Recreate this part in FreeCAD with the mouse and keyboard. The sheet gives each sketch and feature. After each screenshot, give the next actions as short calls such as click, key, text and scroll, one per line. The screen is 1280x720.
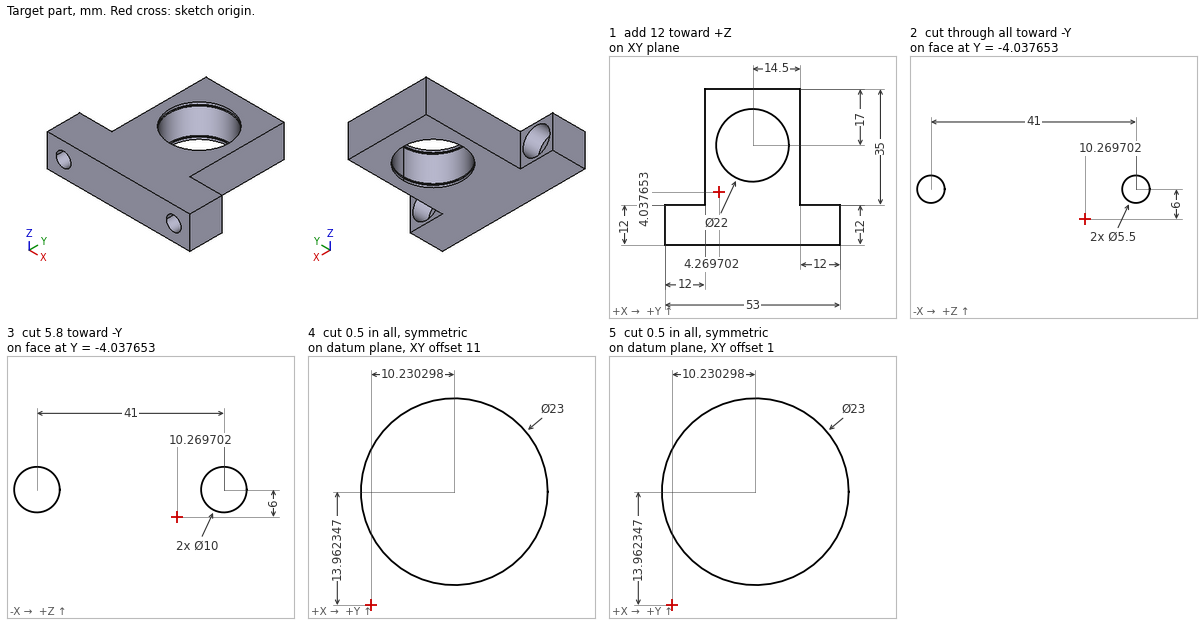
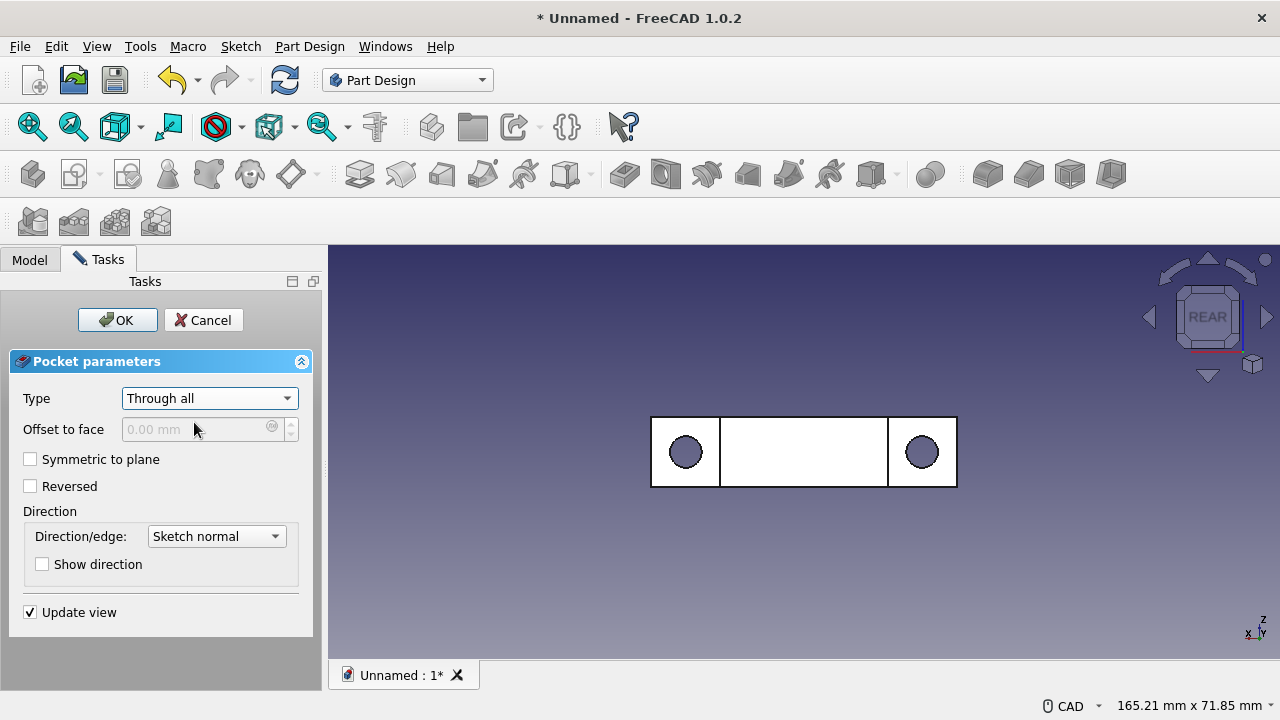
click(118, 320)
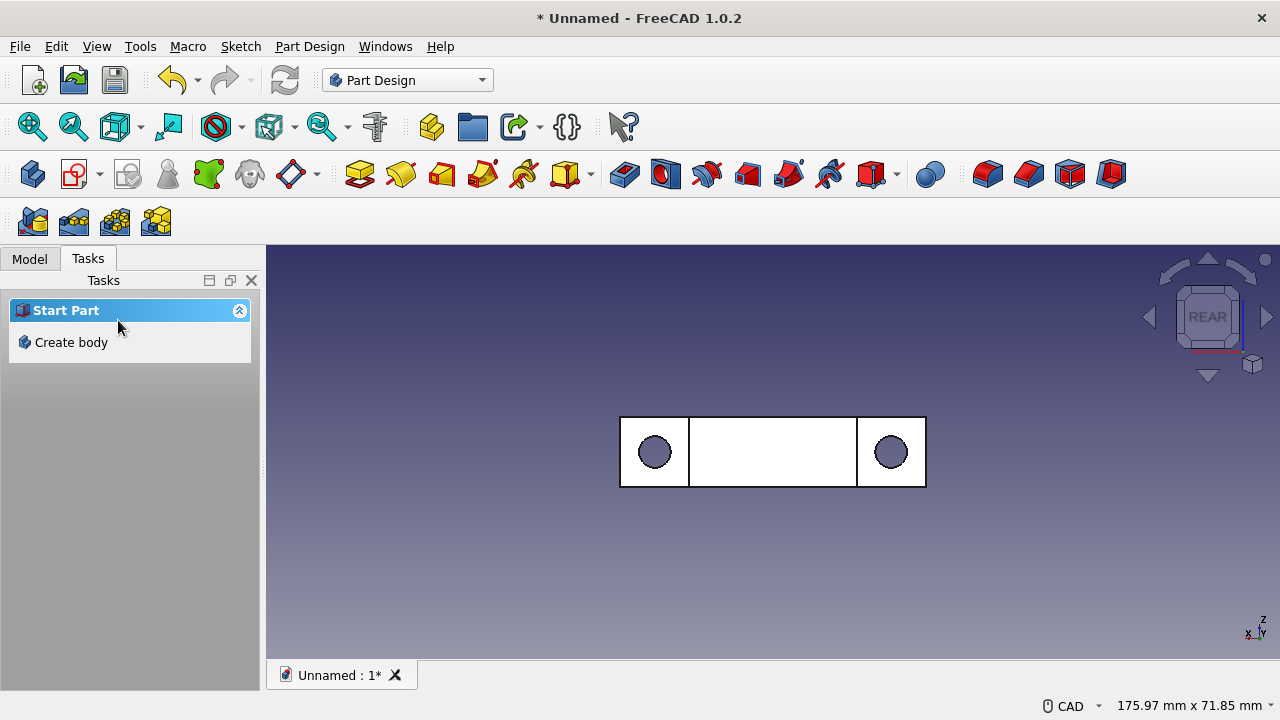
click(33, 128)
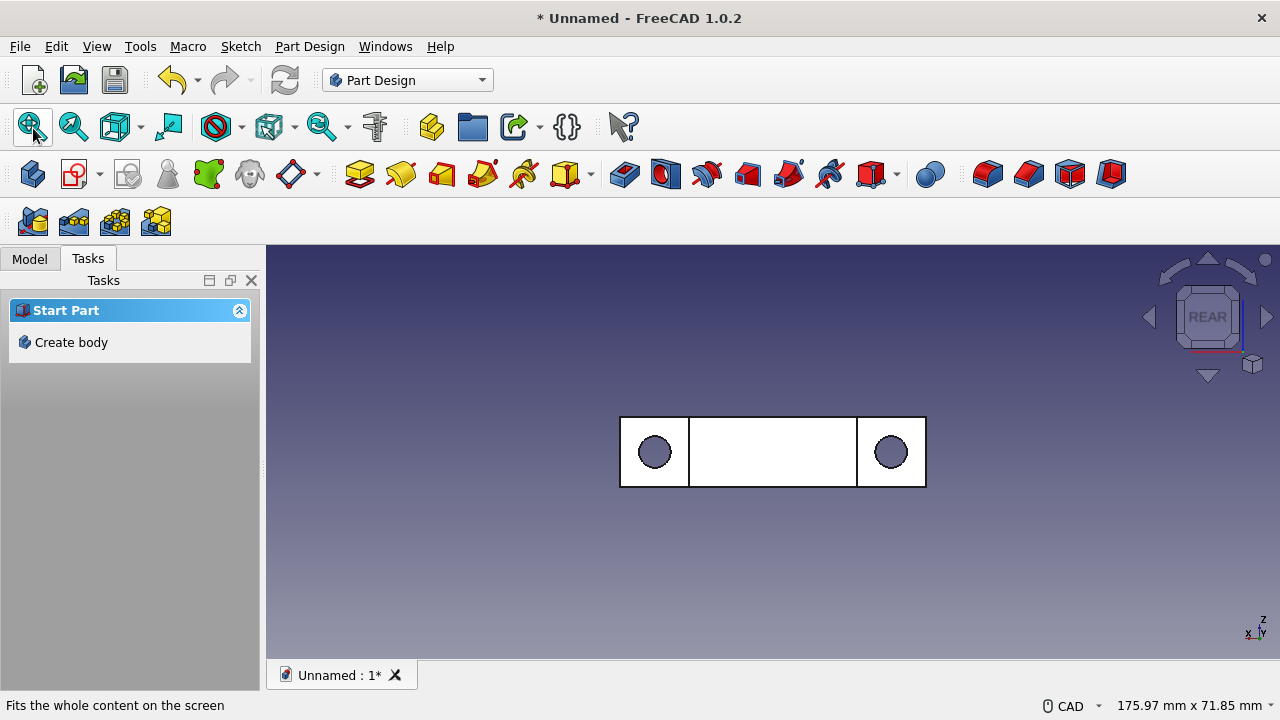
click(675, 471)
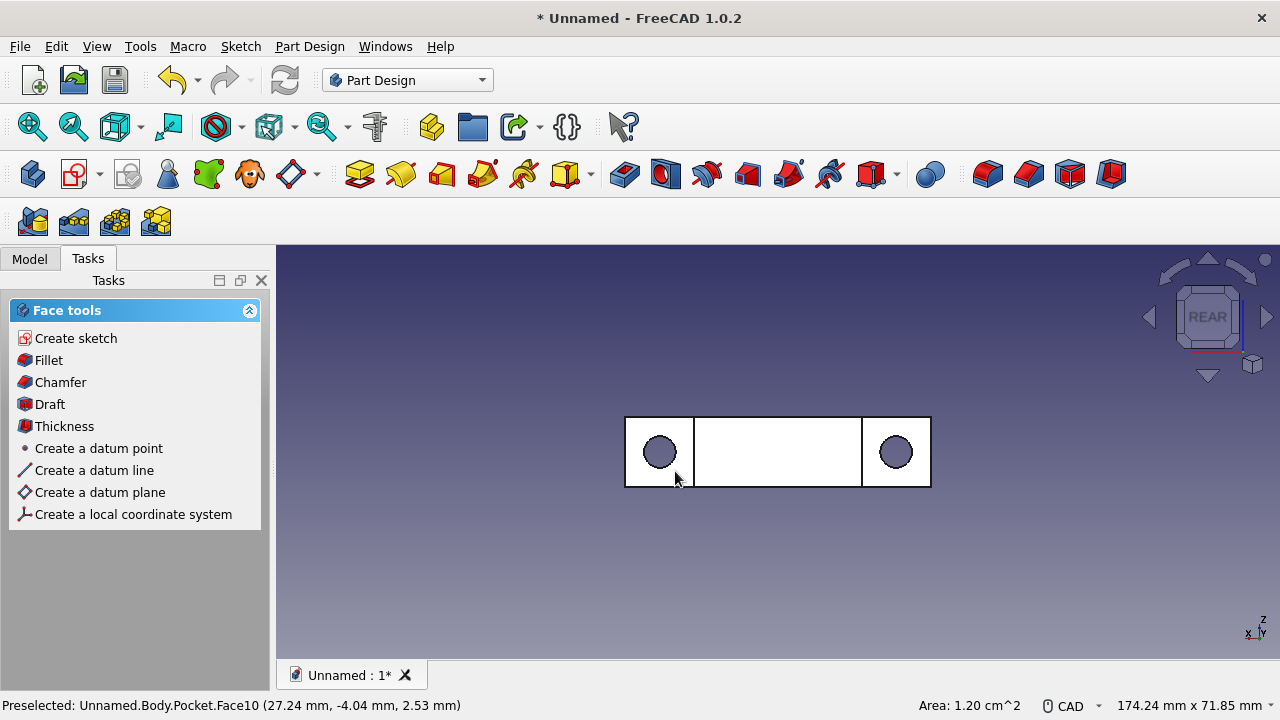
click(74, 174)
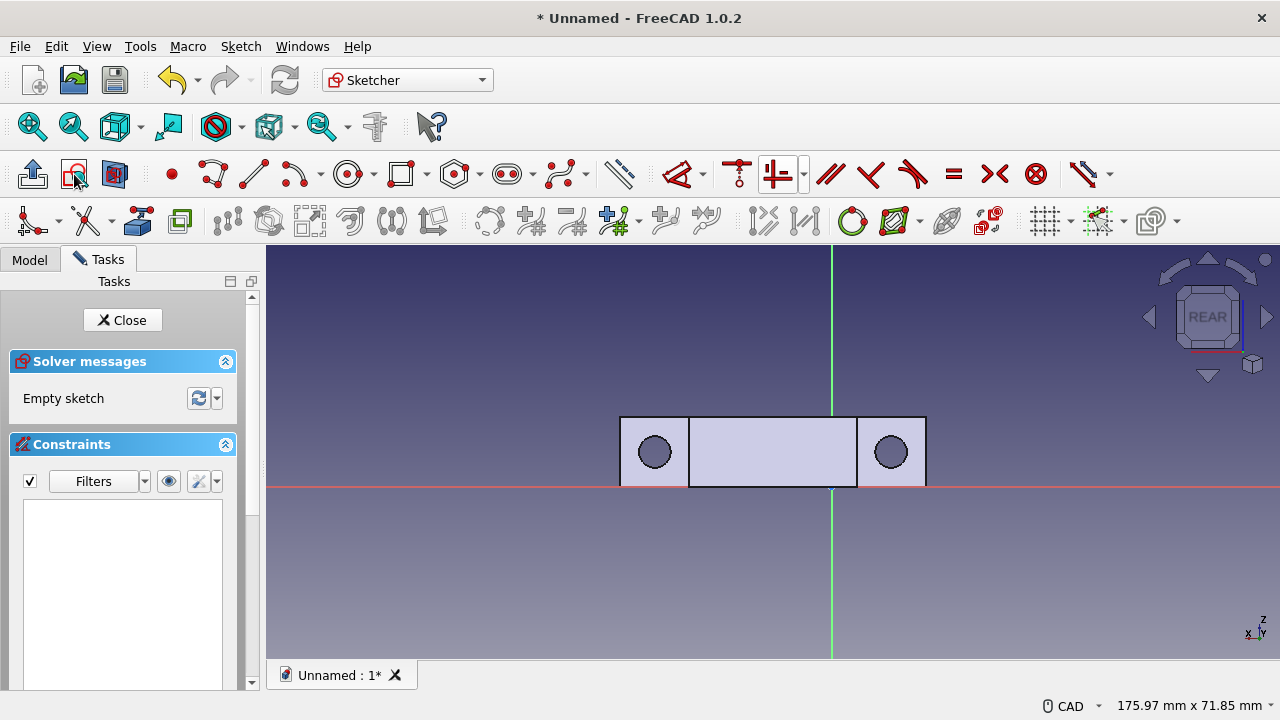
click(115, 174)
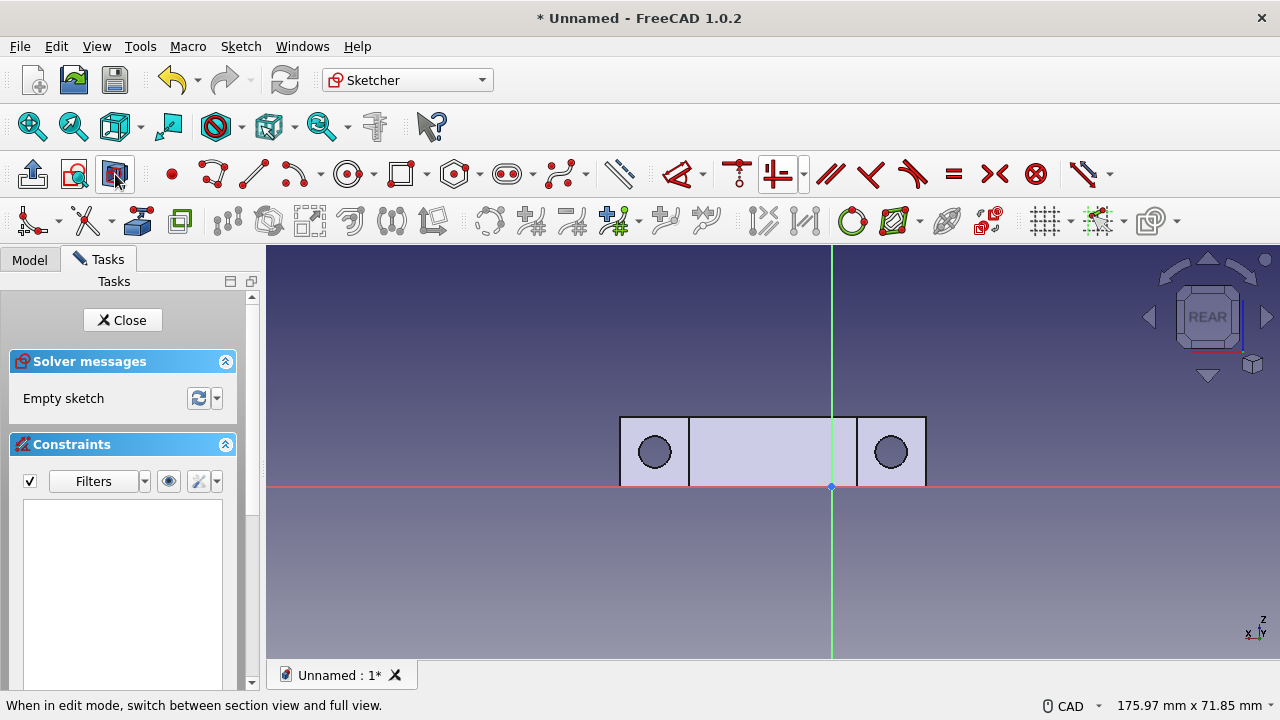
scroll(856, 458, up, 3)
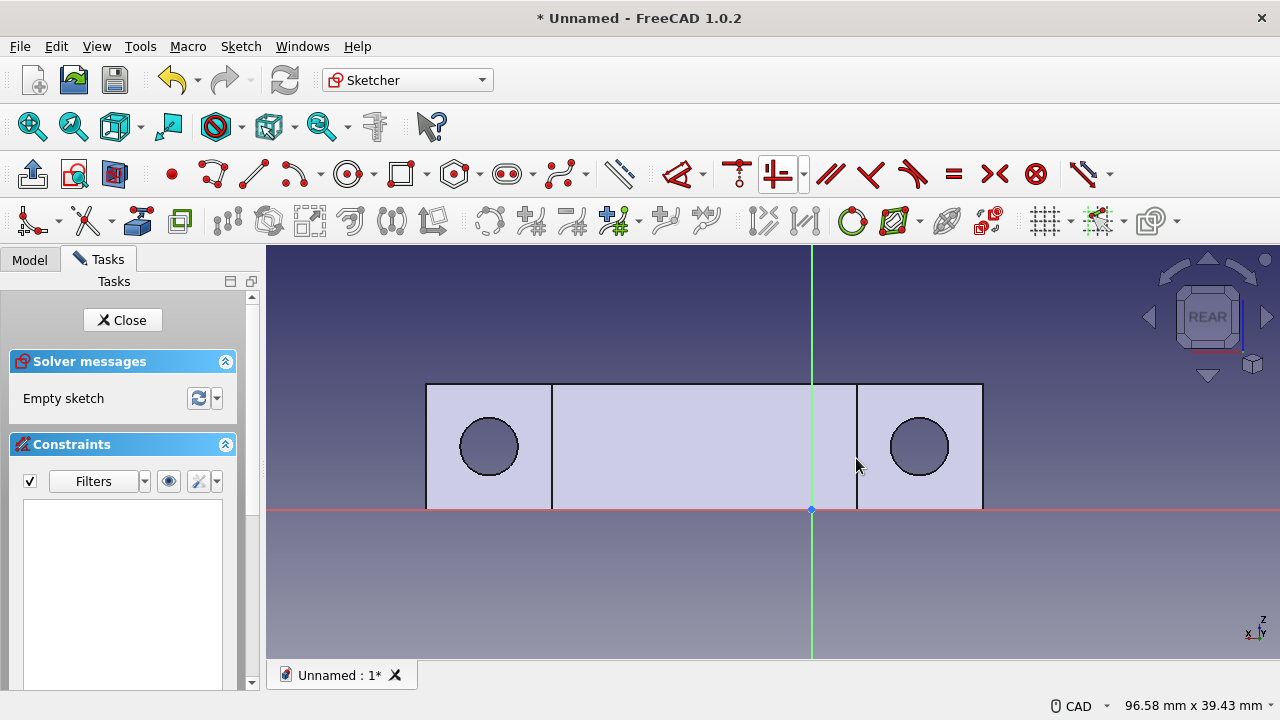
click(348, 174)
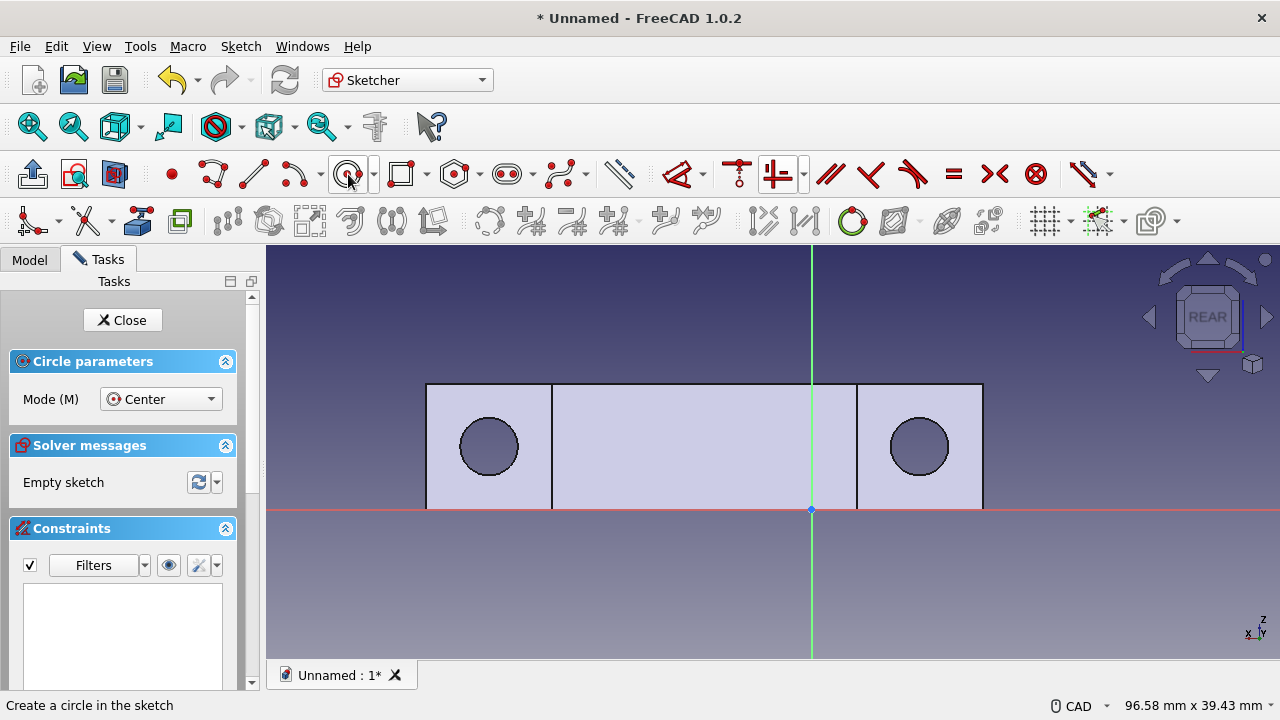
click(920, 447)
click(957, 410)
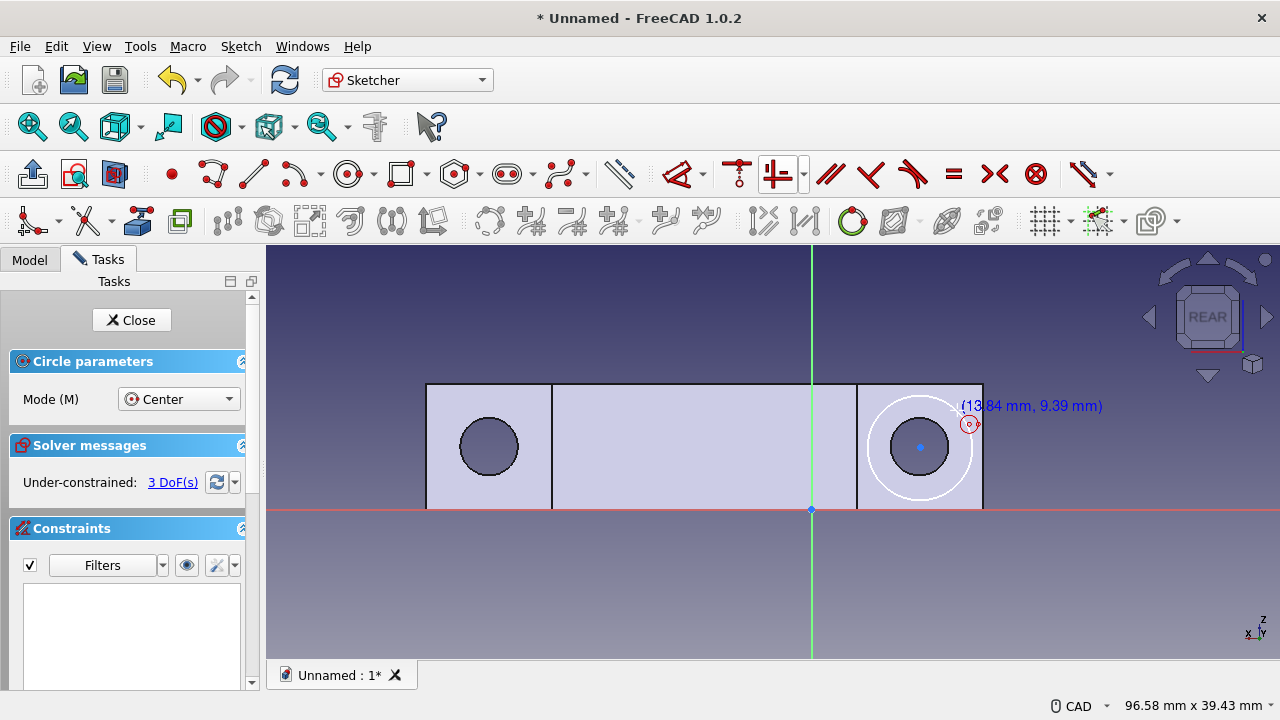
click(489, 447)
click(526, 410)
key(Escape)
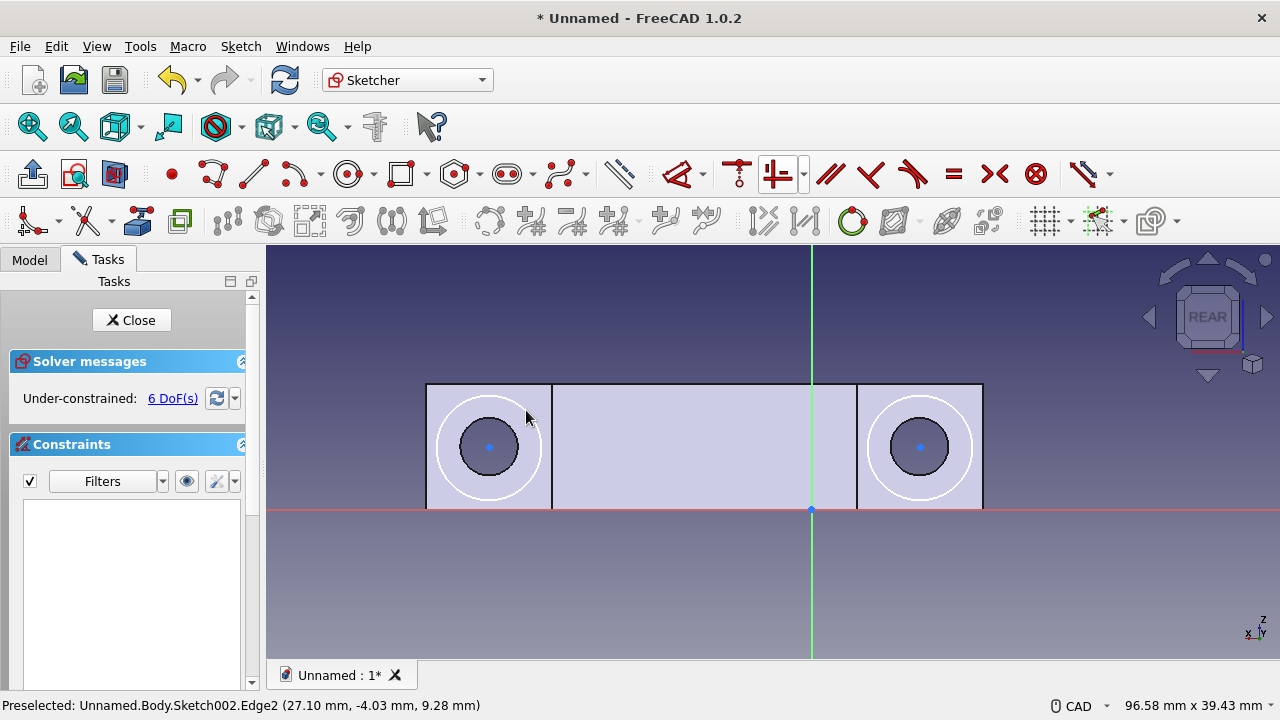
click(957, 411)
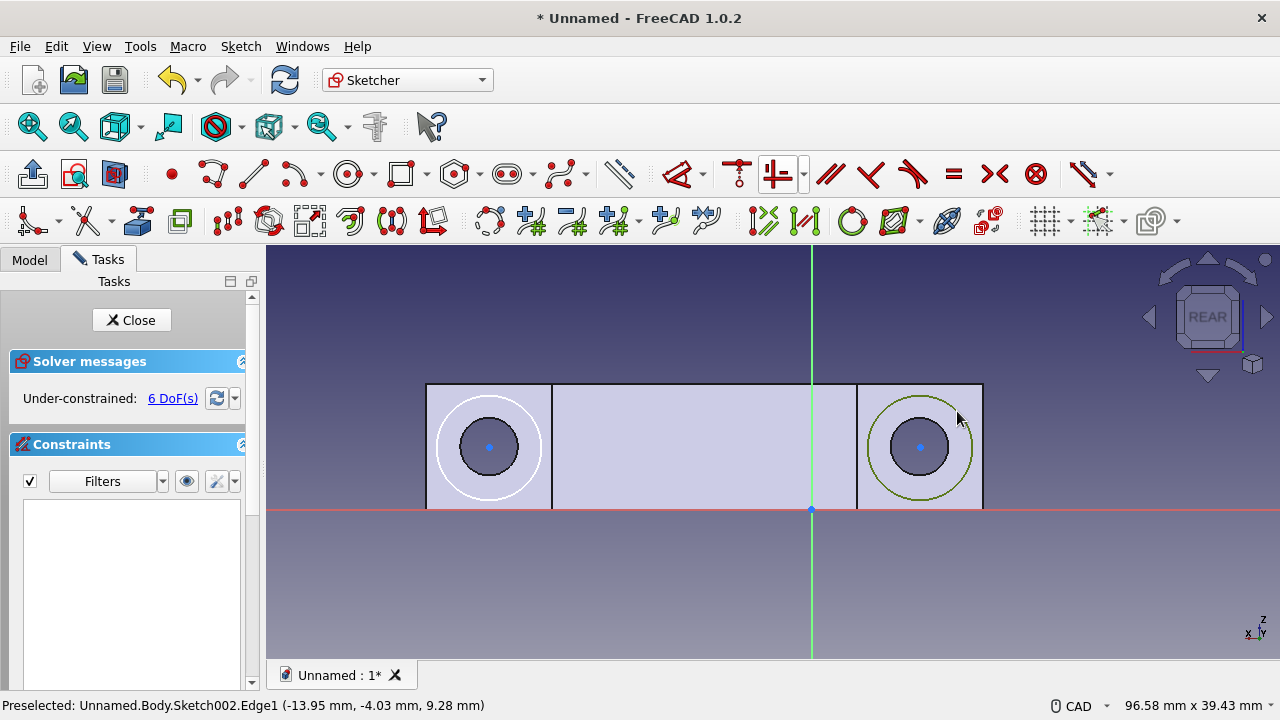
click(526, 411)